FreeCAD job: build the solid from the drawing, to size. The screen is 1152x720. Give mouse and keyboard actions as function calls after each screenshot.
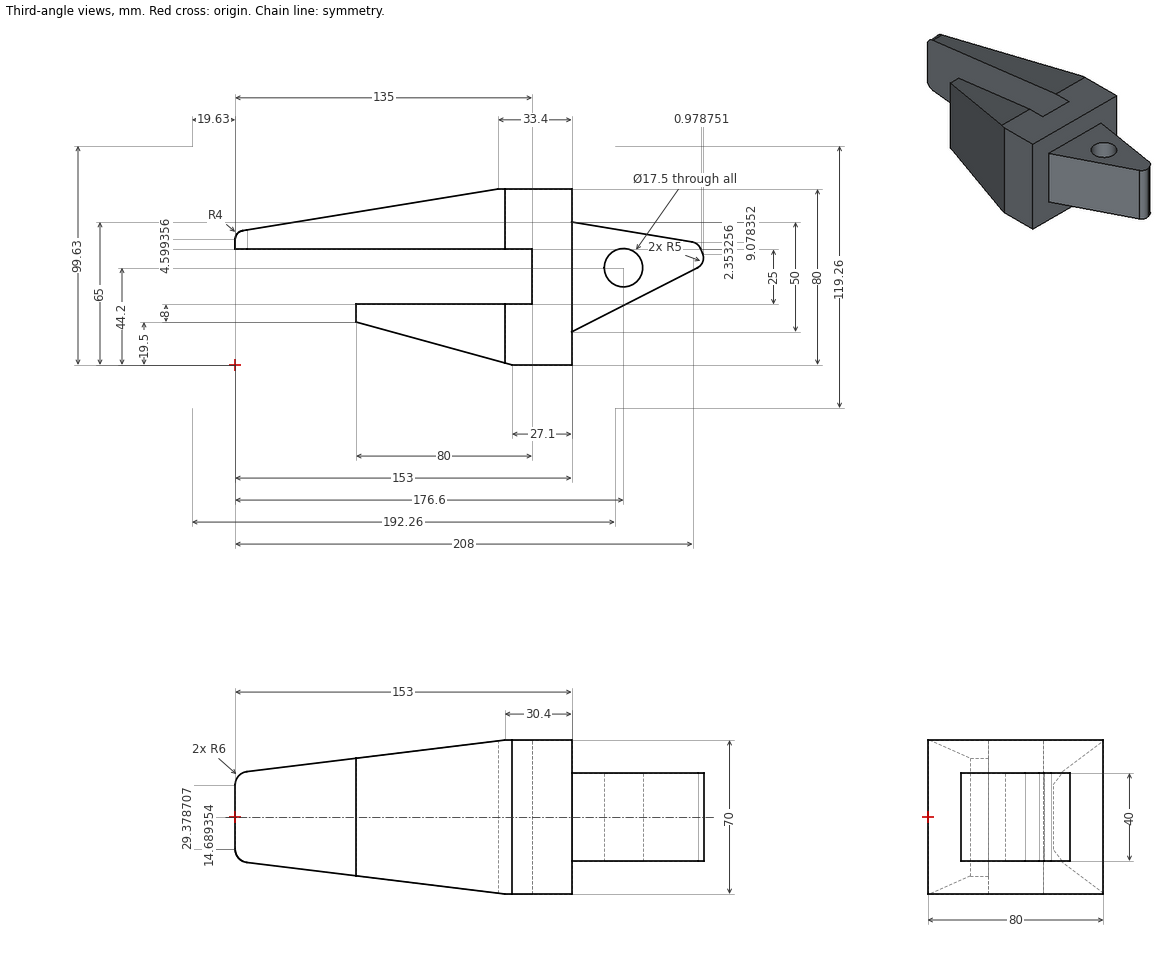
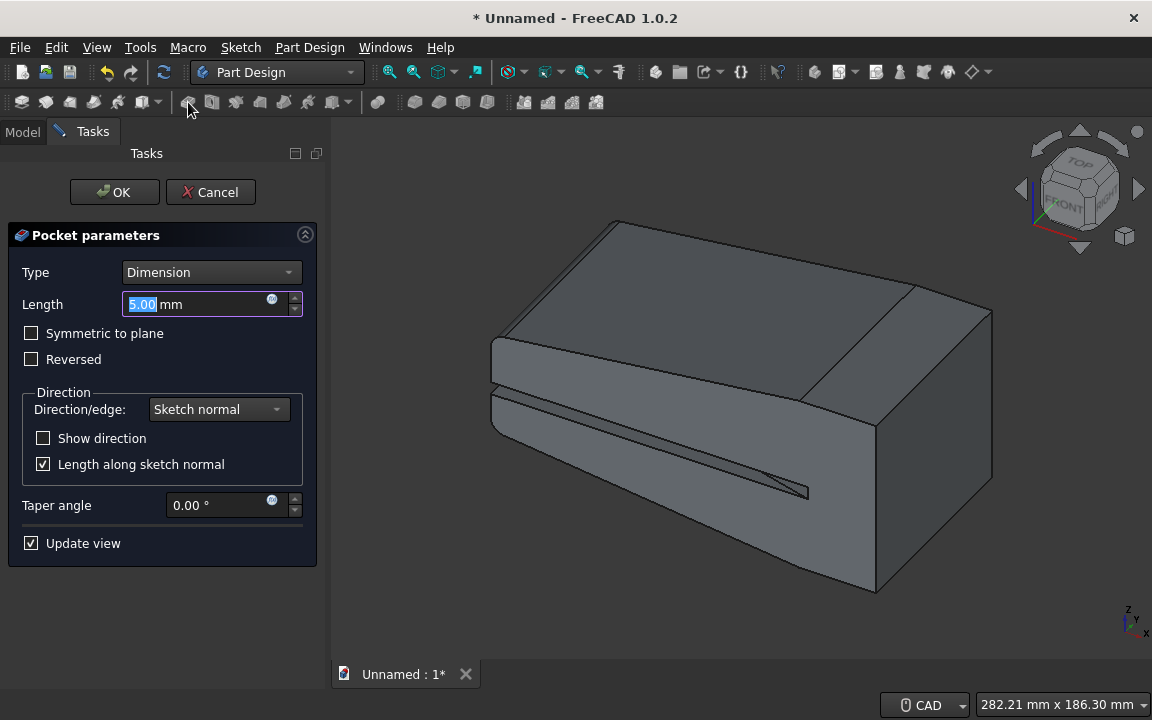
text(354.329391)
key(Tab)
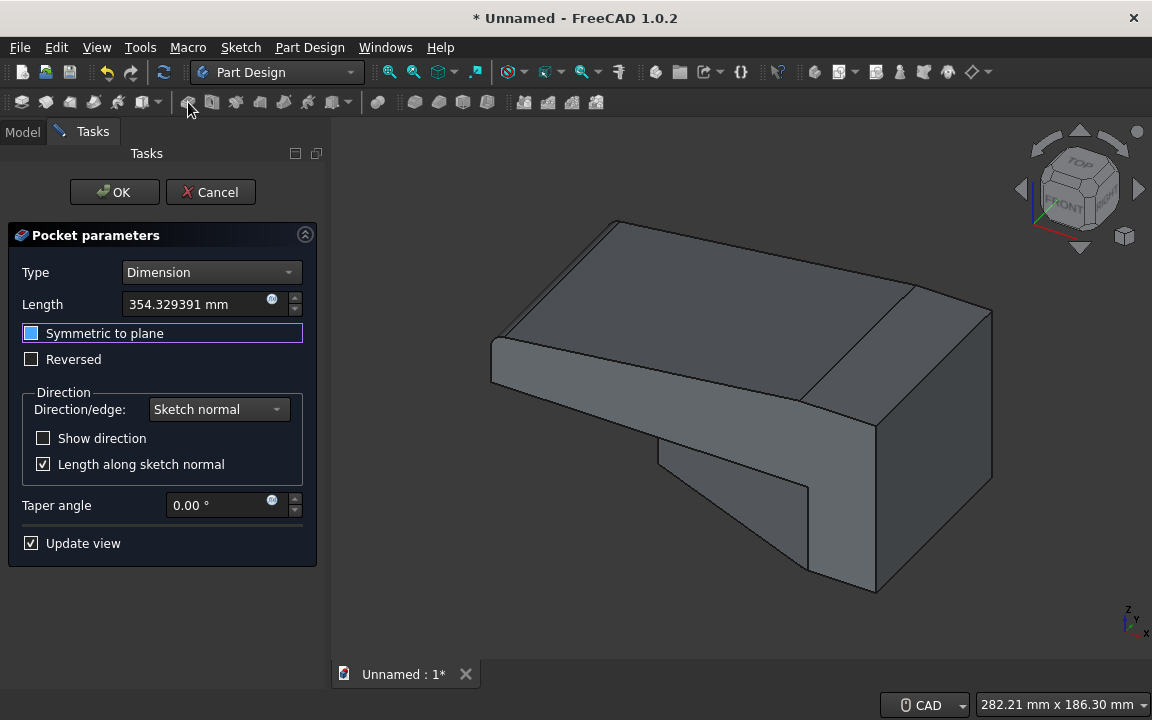
click(30, 333)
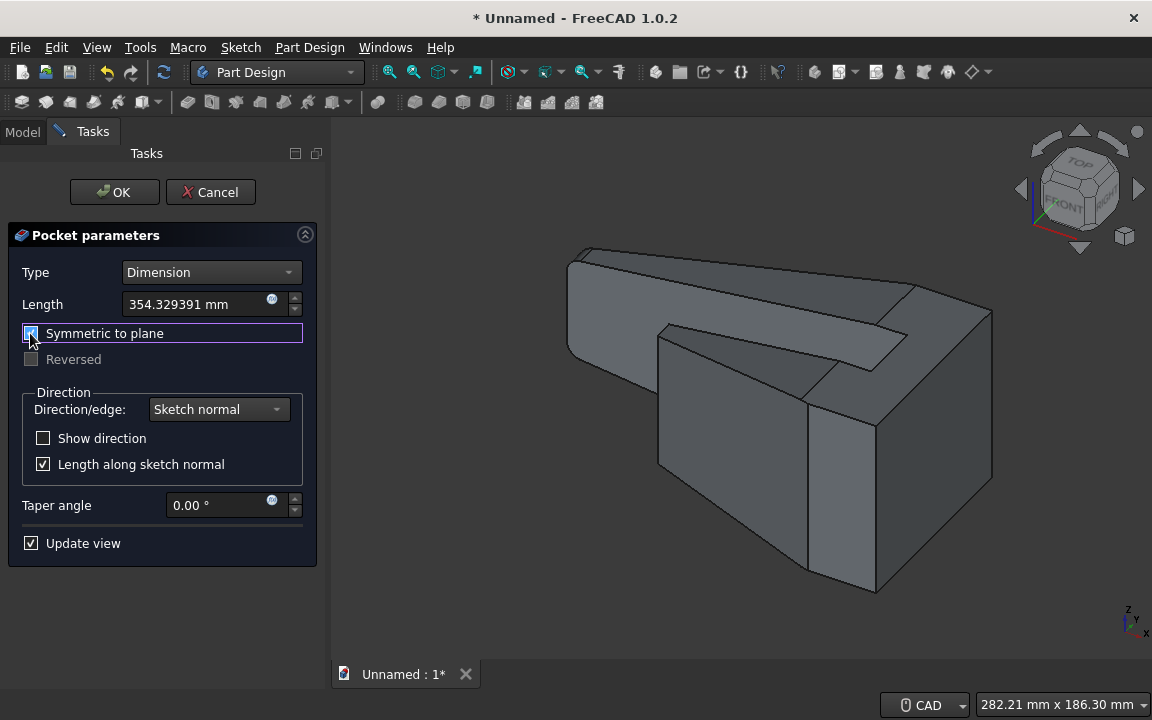
click(115, 192)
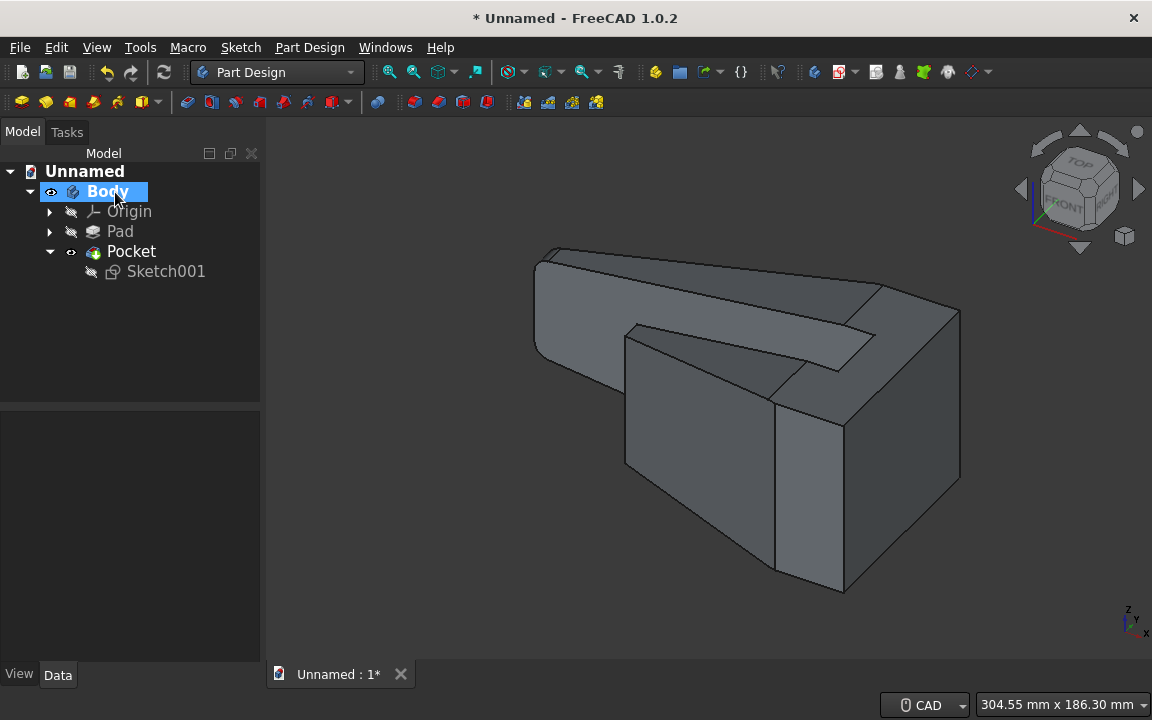
click(840, 72)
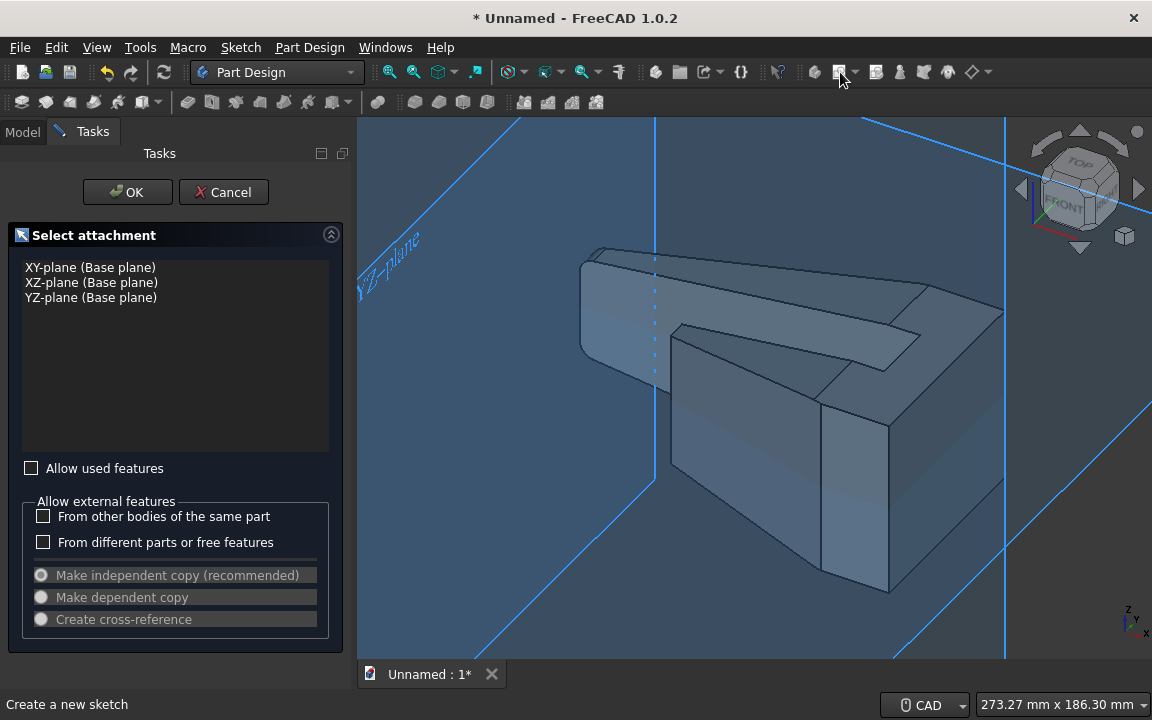
click(82, 268)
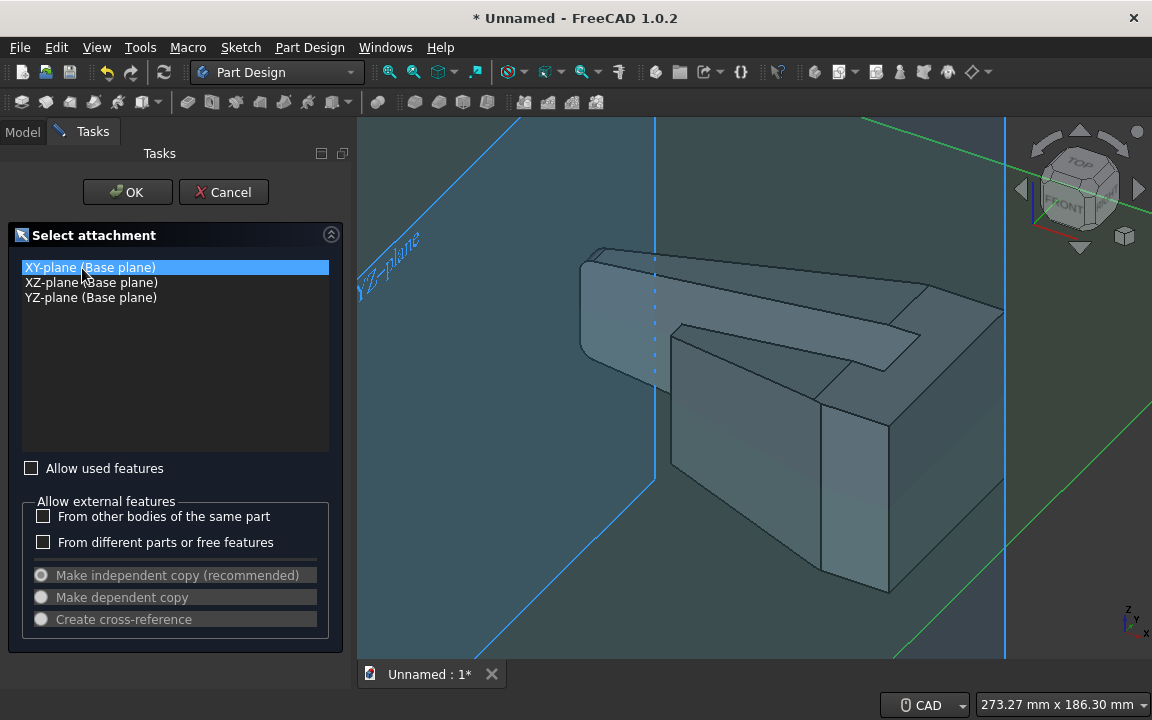
click(128, 192)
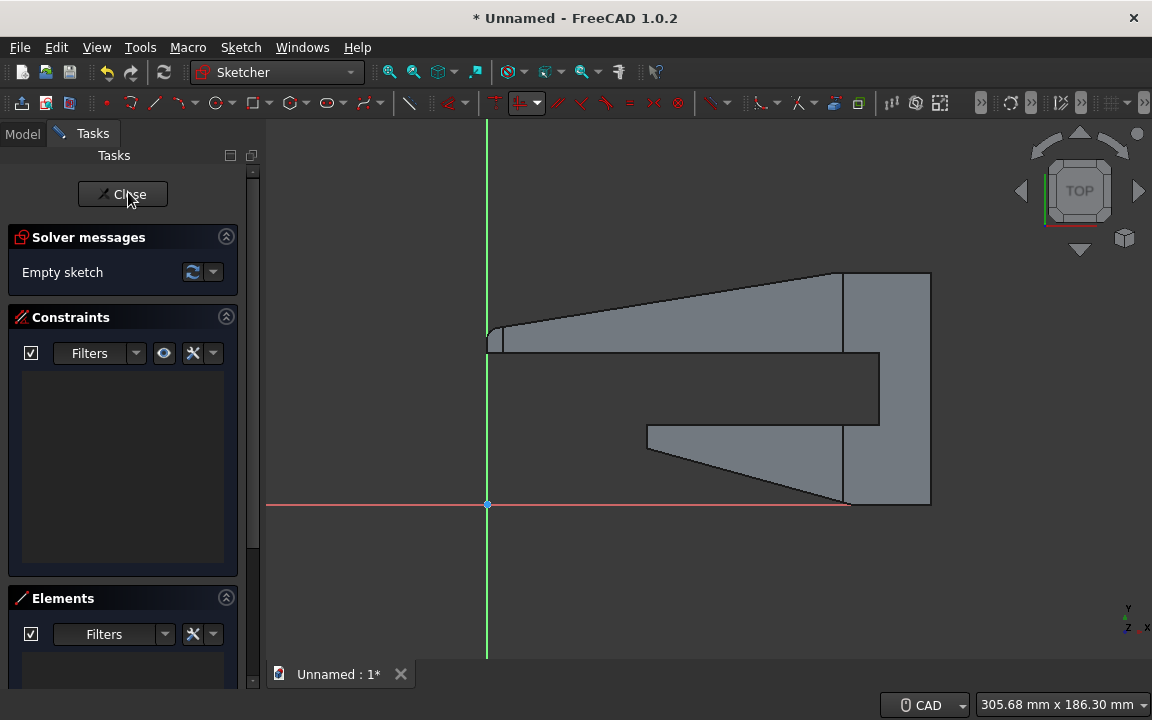
key(q)
key(s)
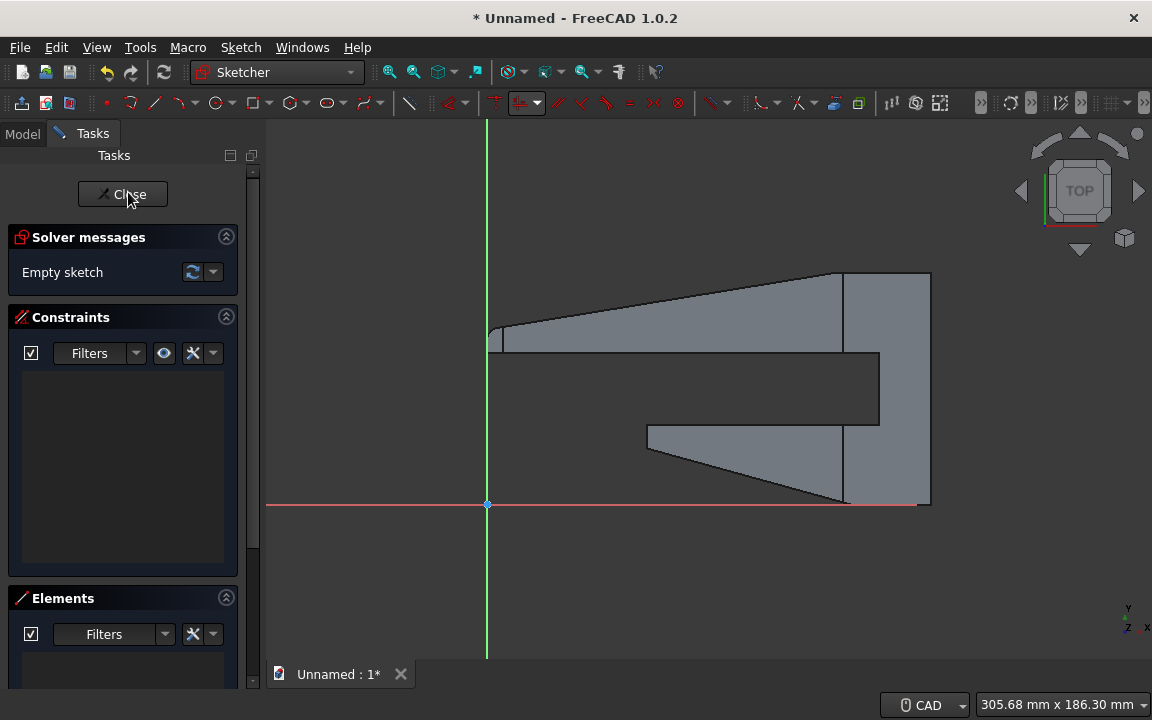
scroll(640, 389, down, 5)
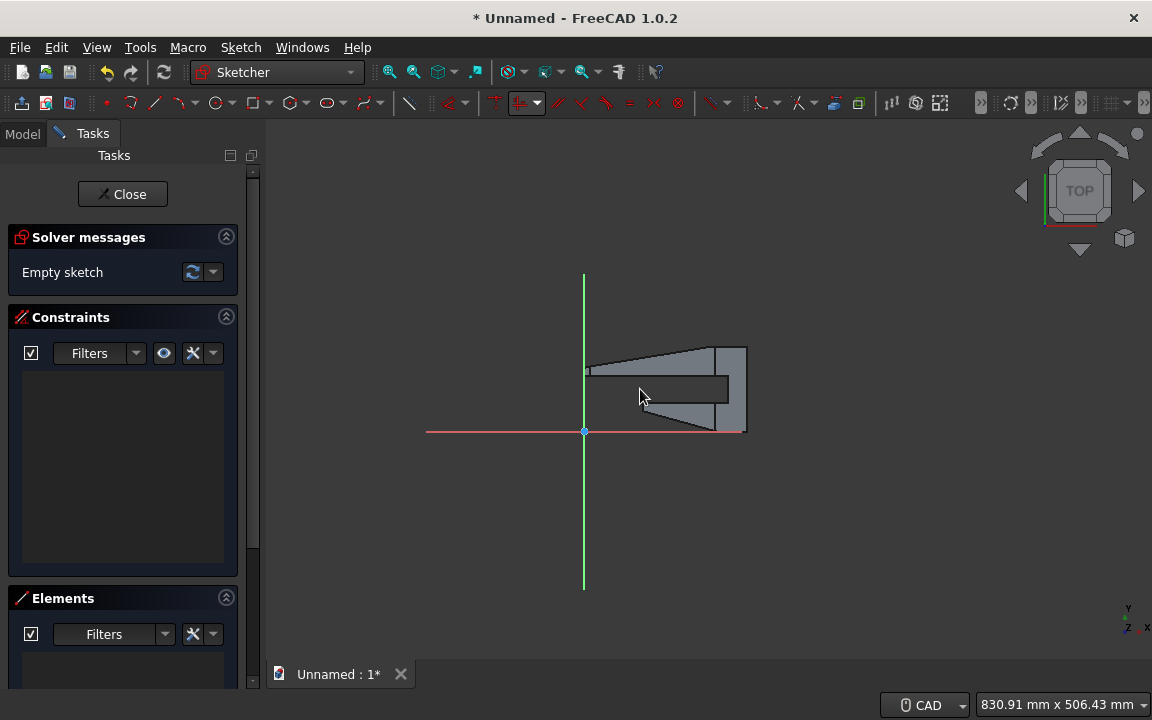
scroll(806, 389, up, 9)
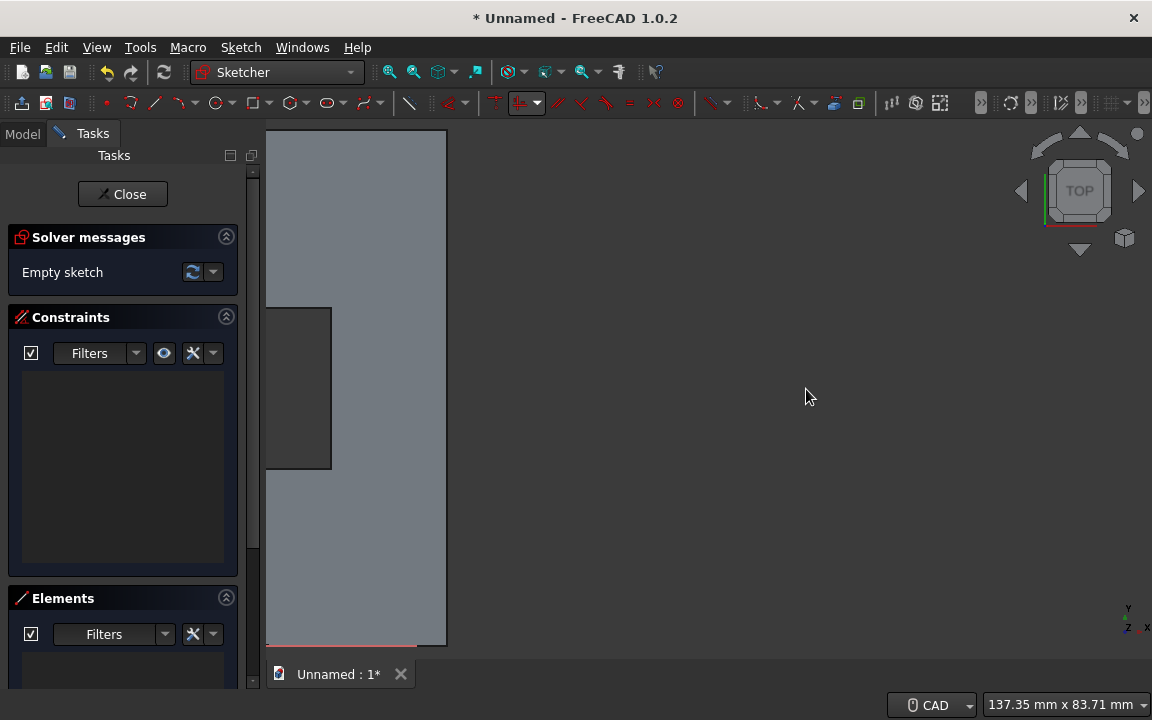
key(g)
key(l)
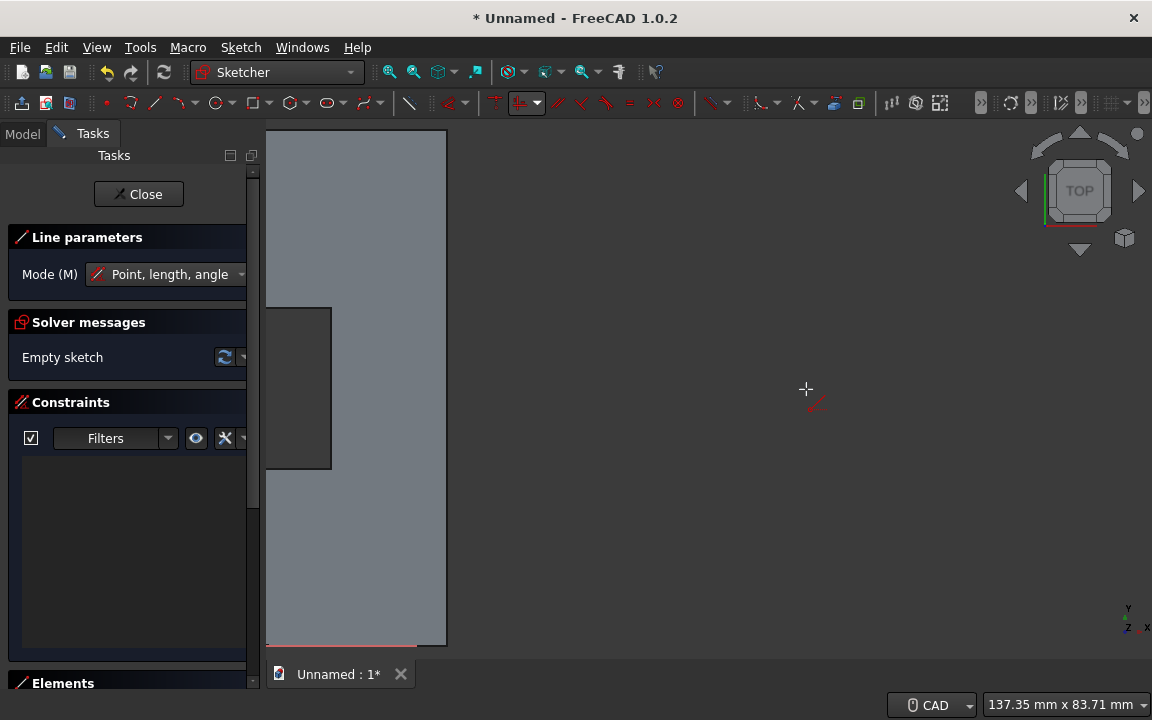
click(832, 320)
click(826, 305)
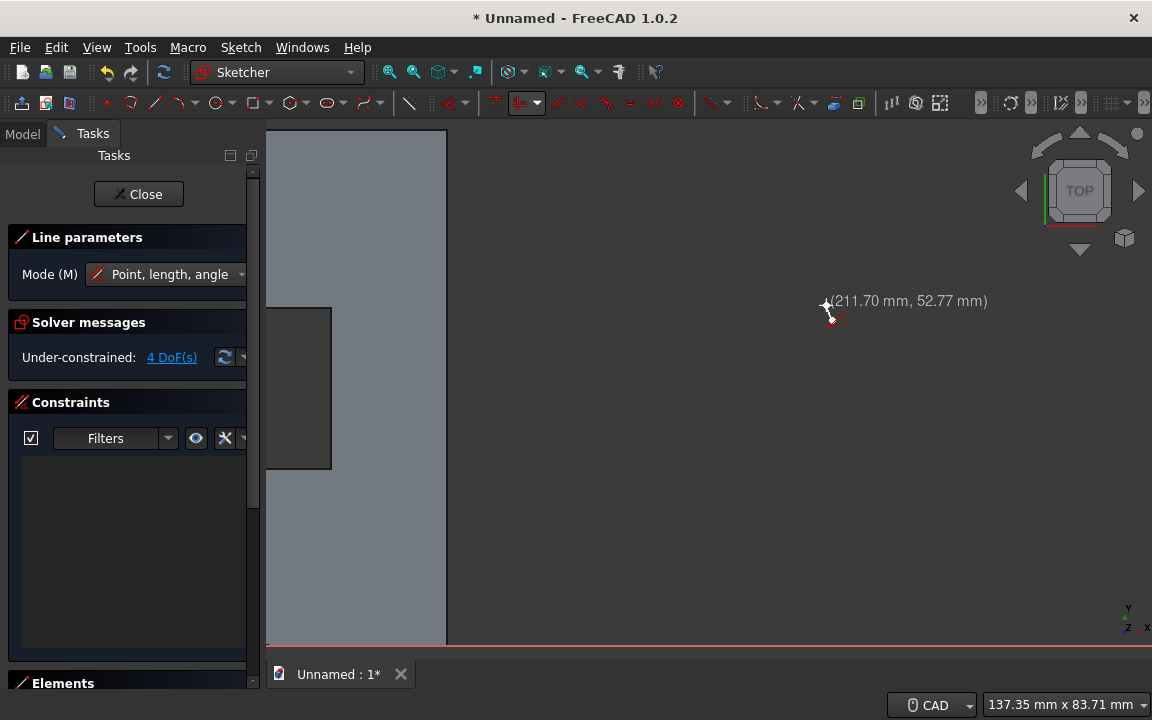
click(132, 104)